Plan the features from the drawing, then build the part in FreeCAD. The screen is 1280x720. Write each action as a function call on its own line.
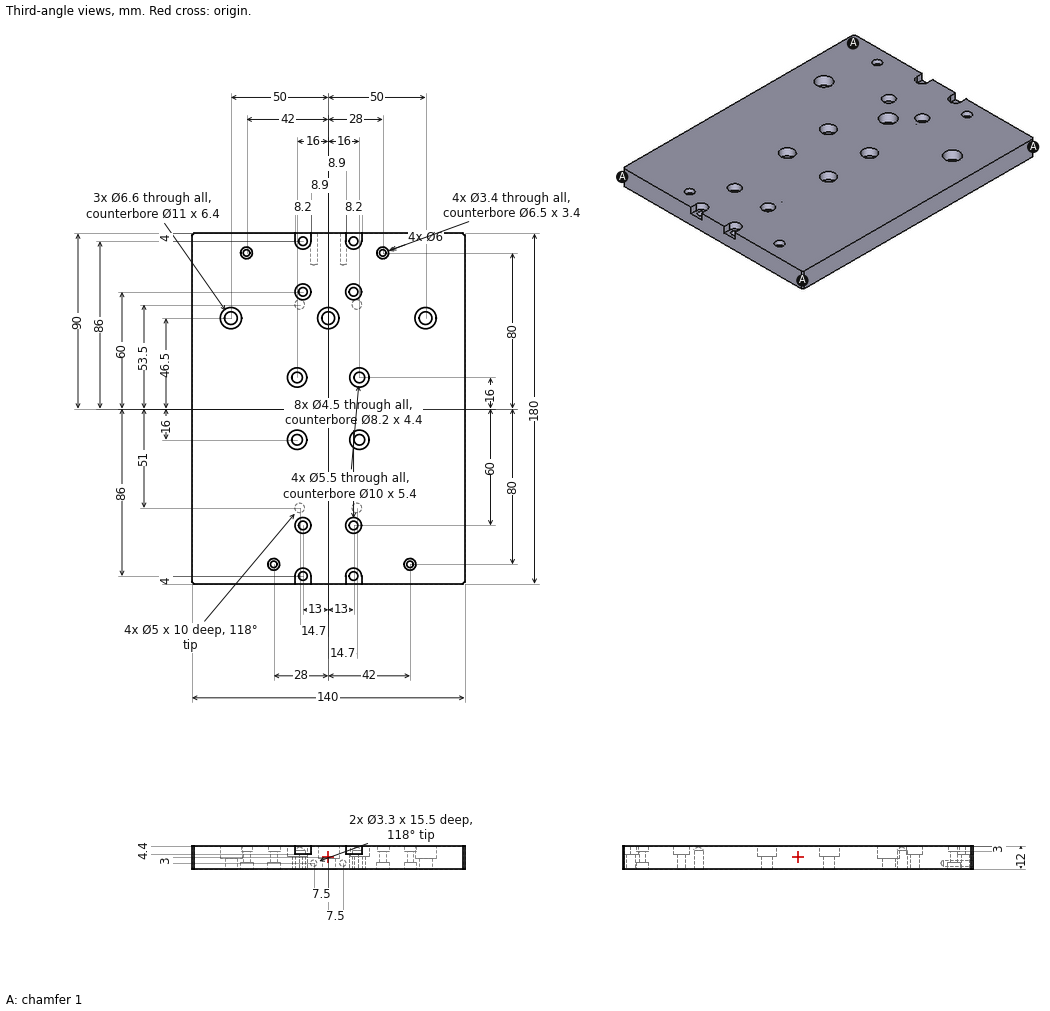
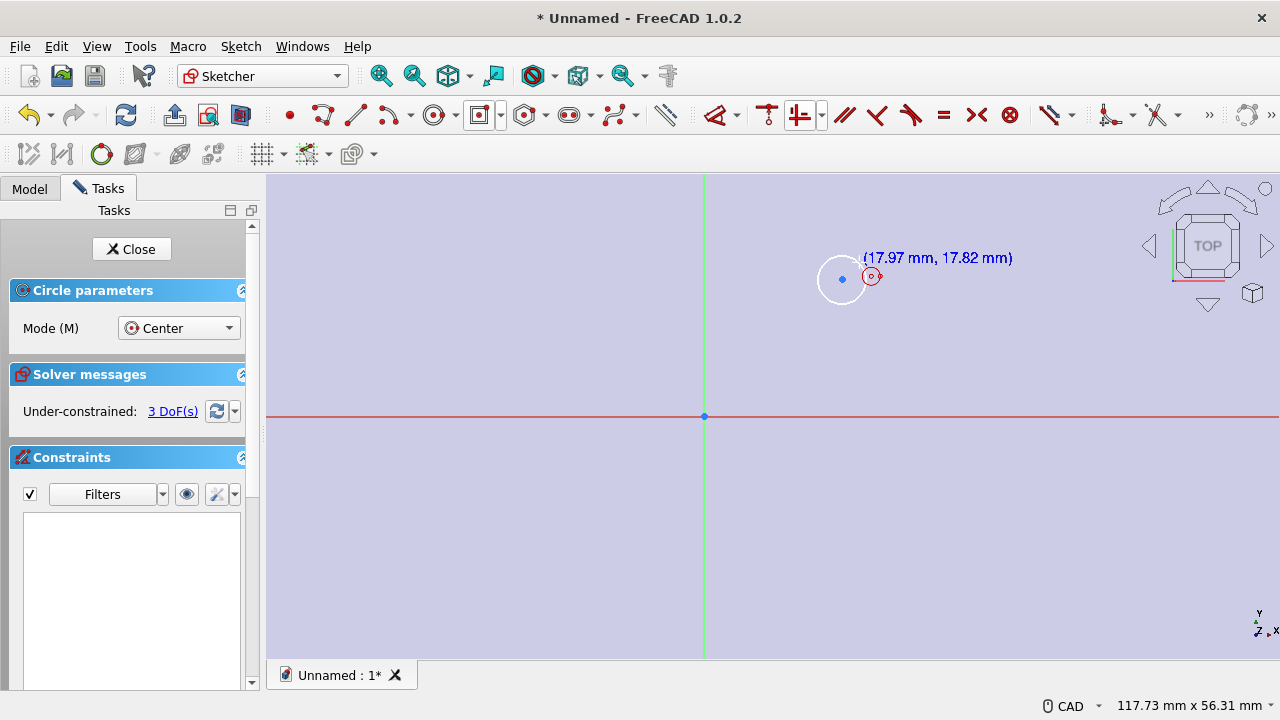
click(566, 279)
click(583, 262)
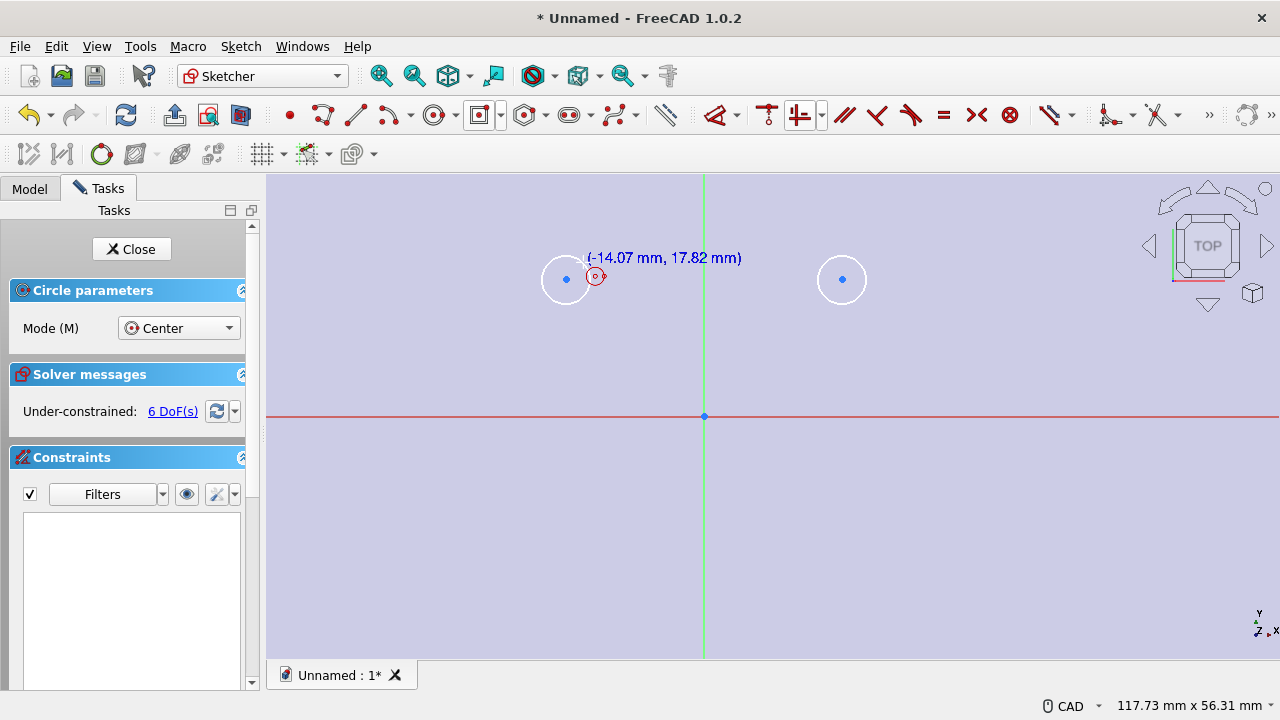
click(566, 554)
click(583, 538)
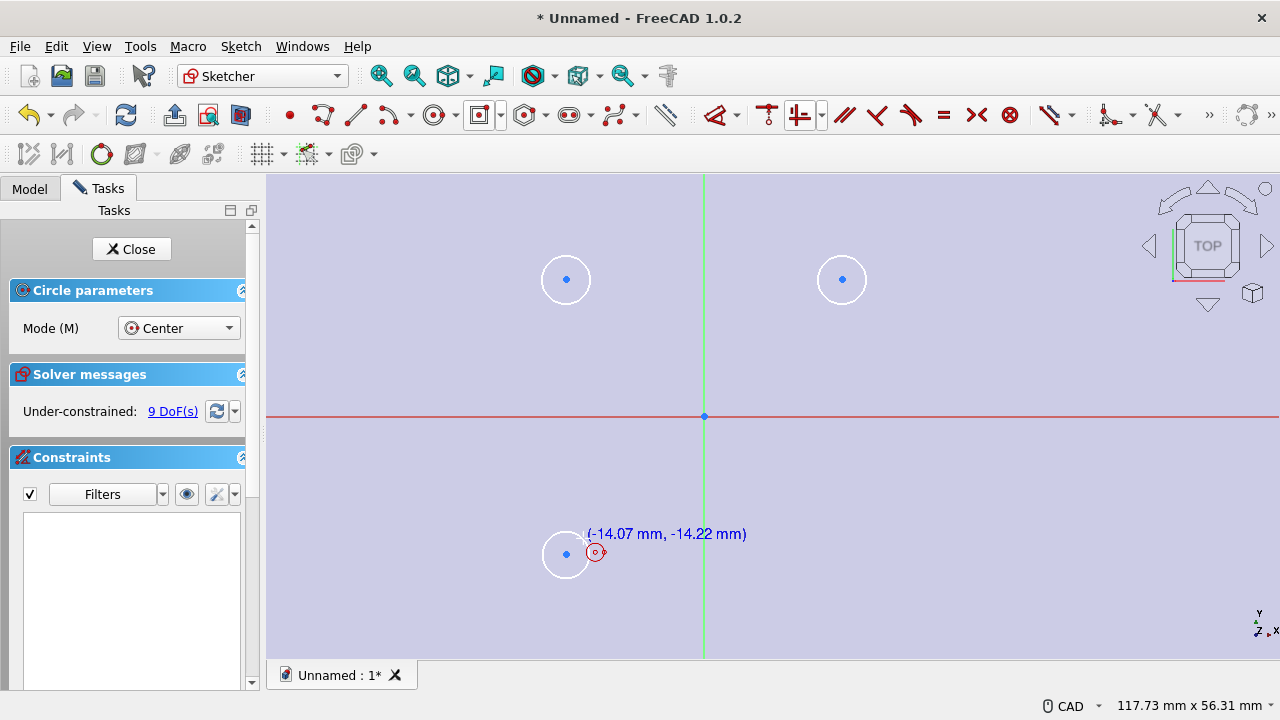
click(842, 554)
click(859, 538)
key(Escape)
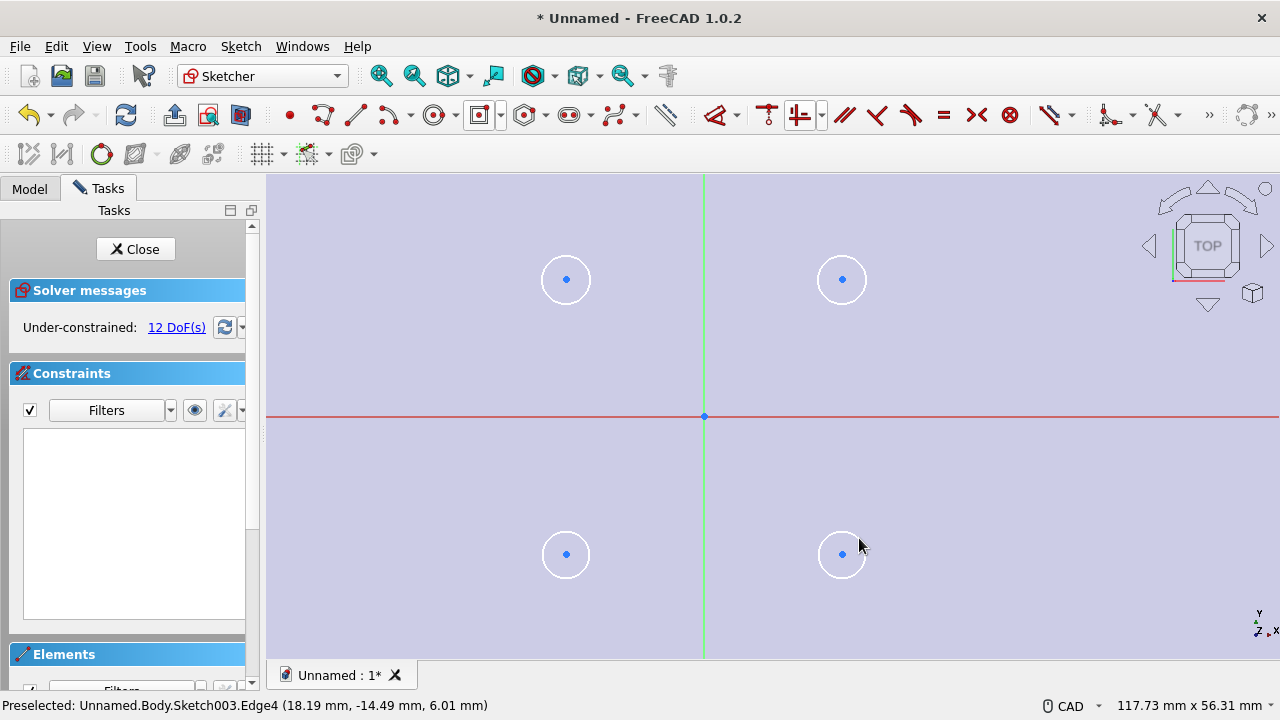
click(859, 263)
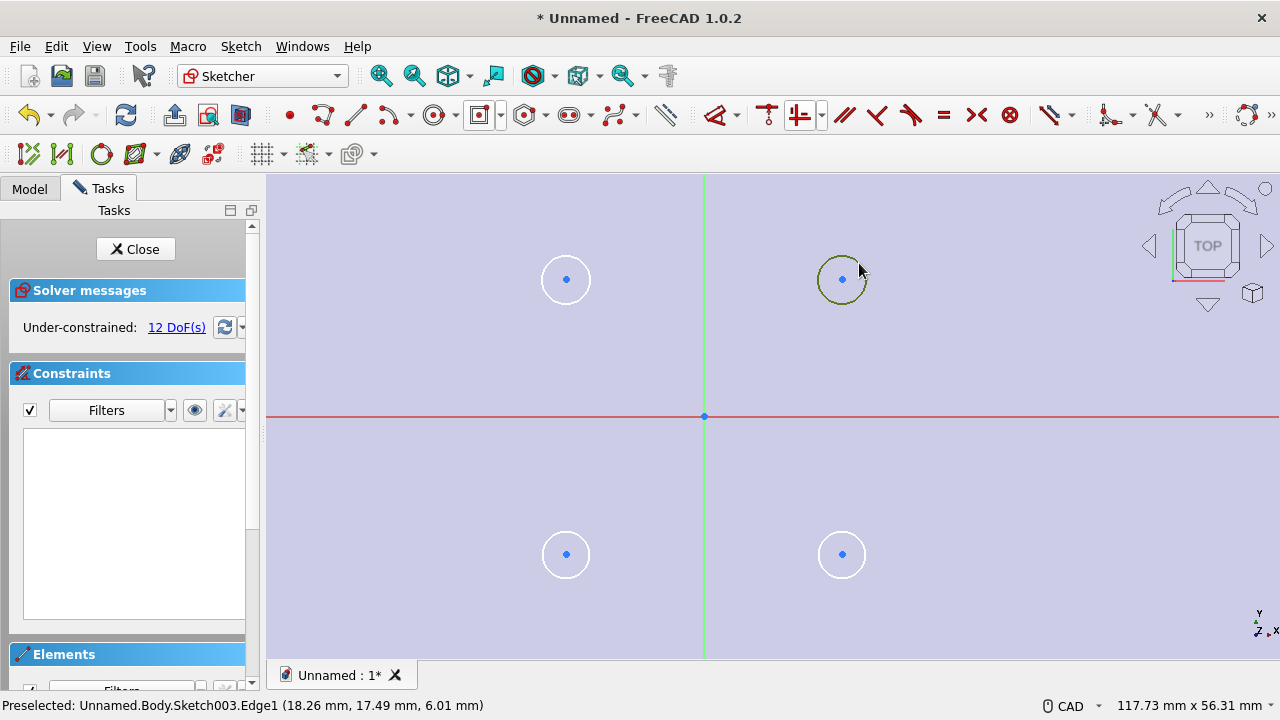
click(583, 263)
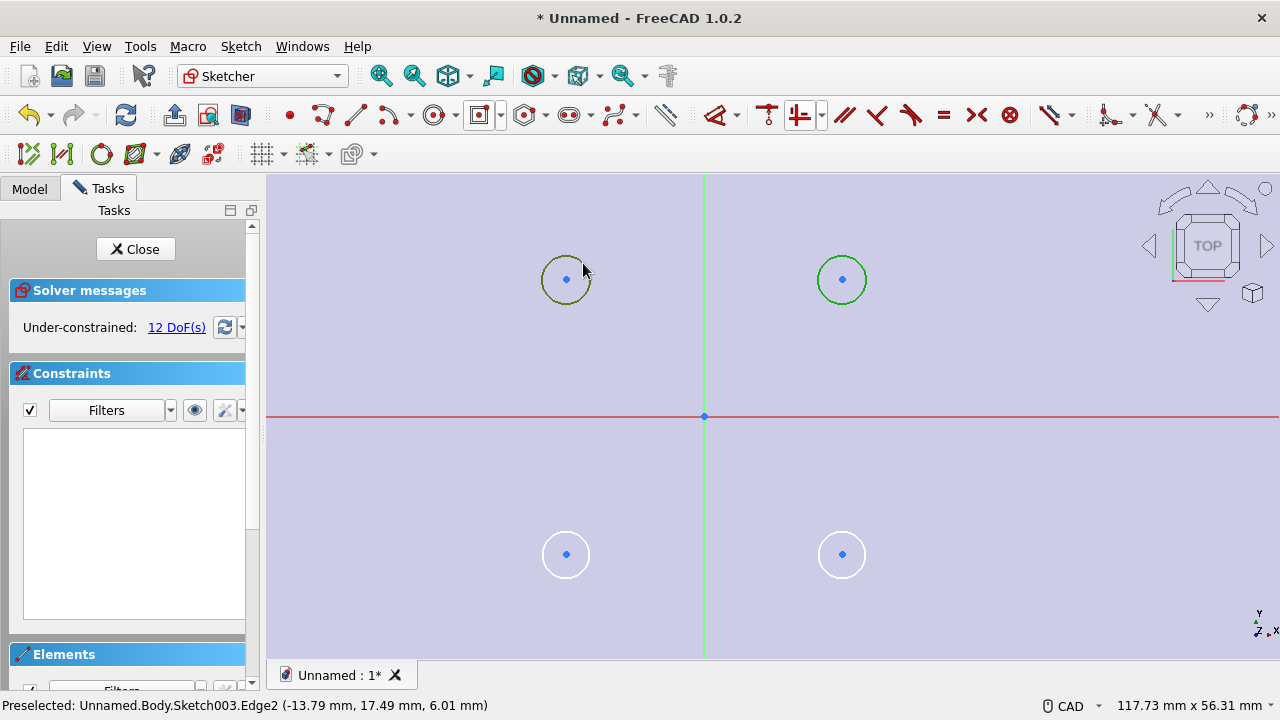
click(582, 538)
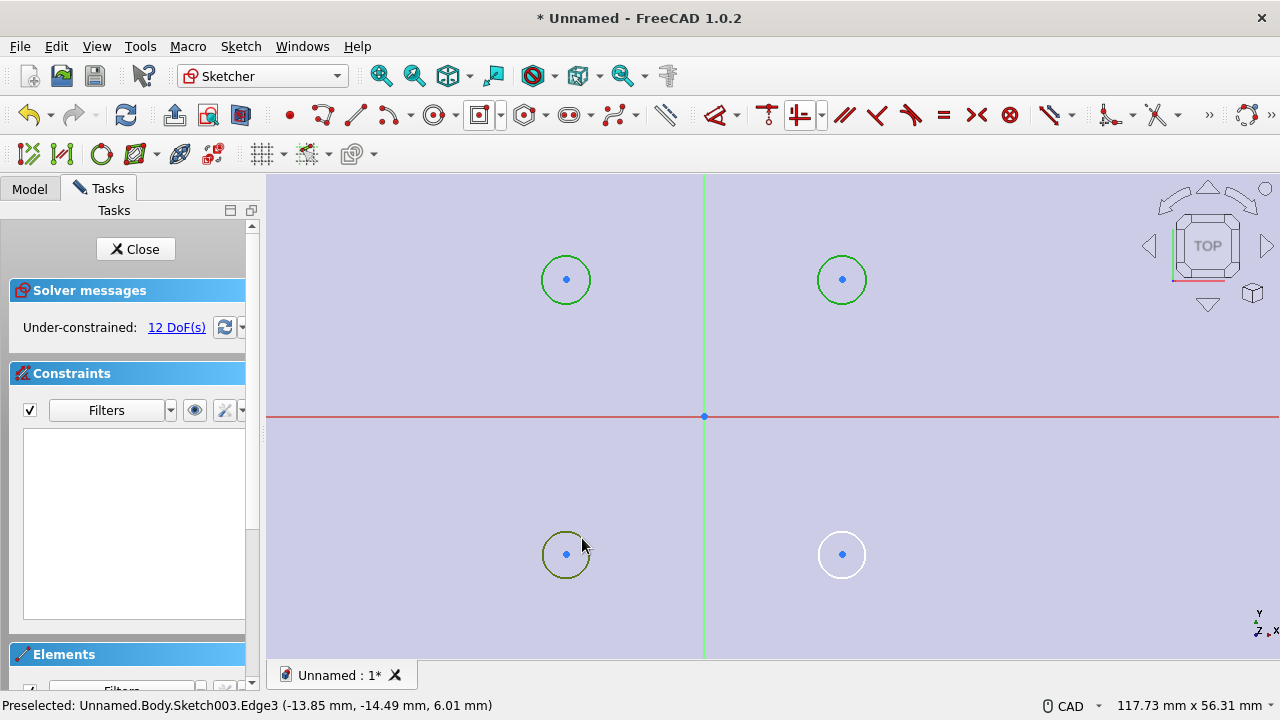
click(858, 538)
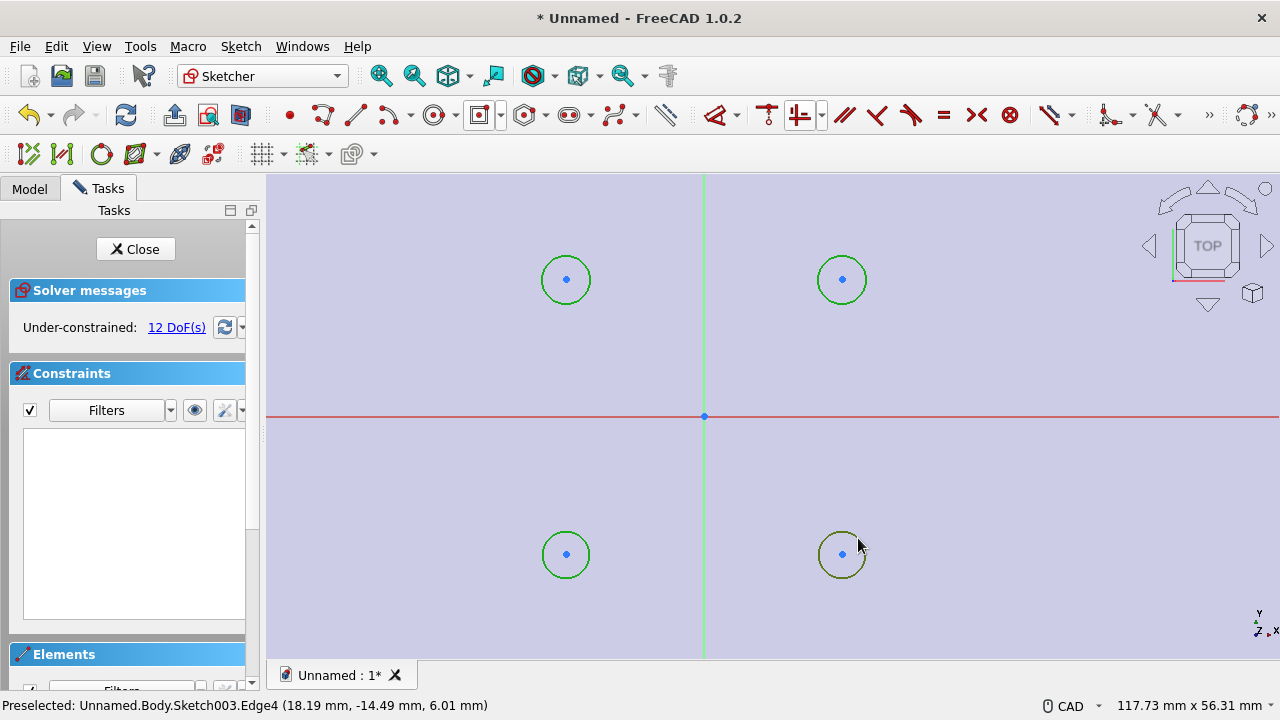
click(944, 116)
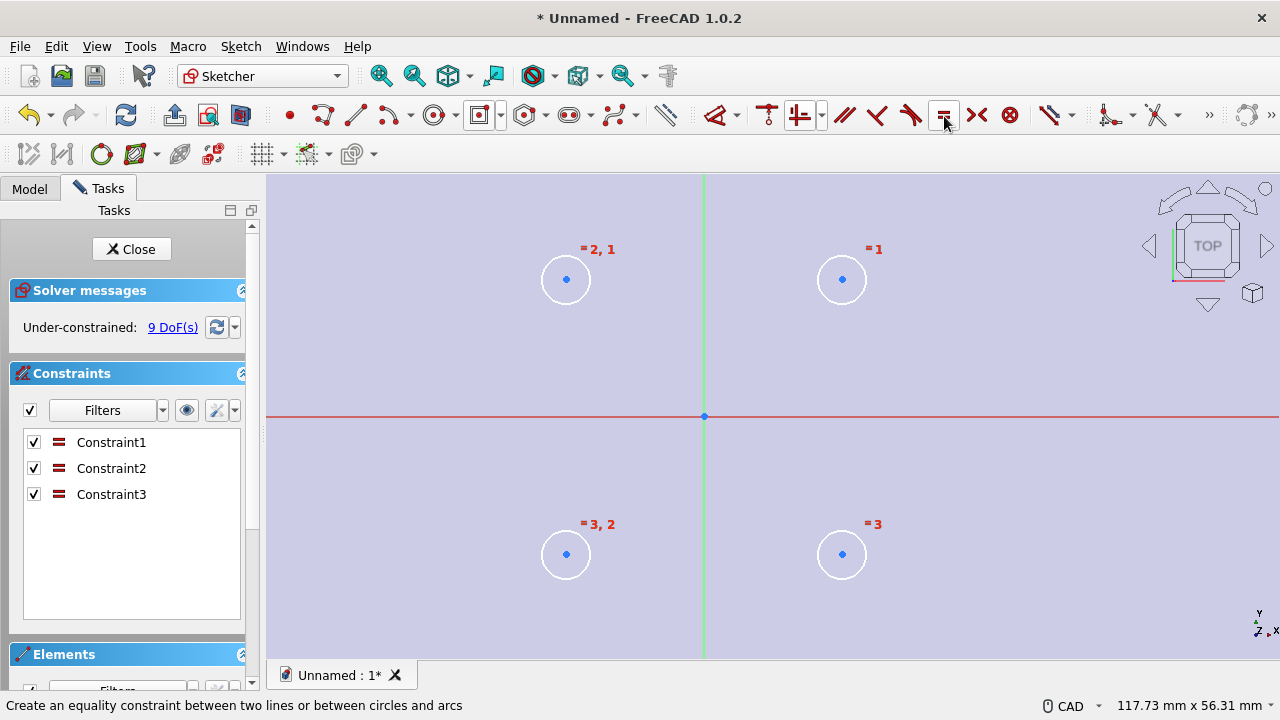
click(714, 116)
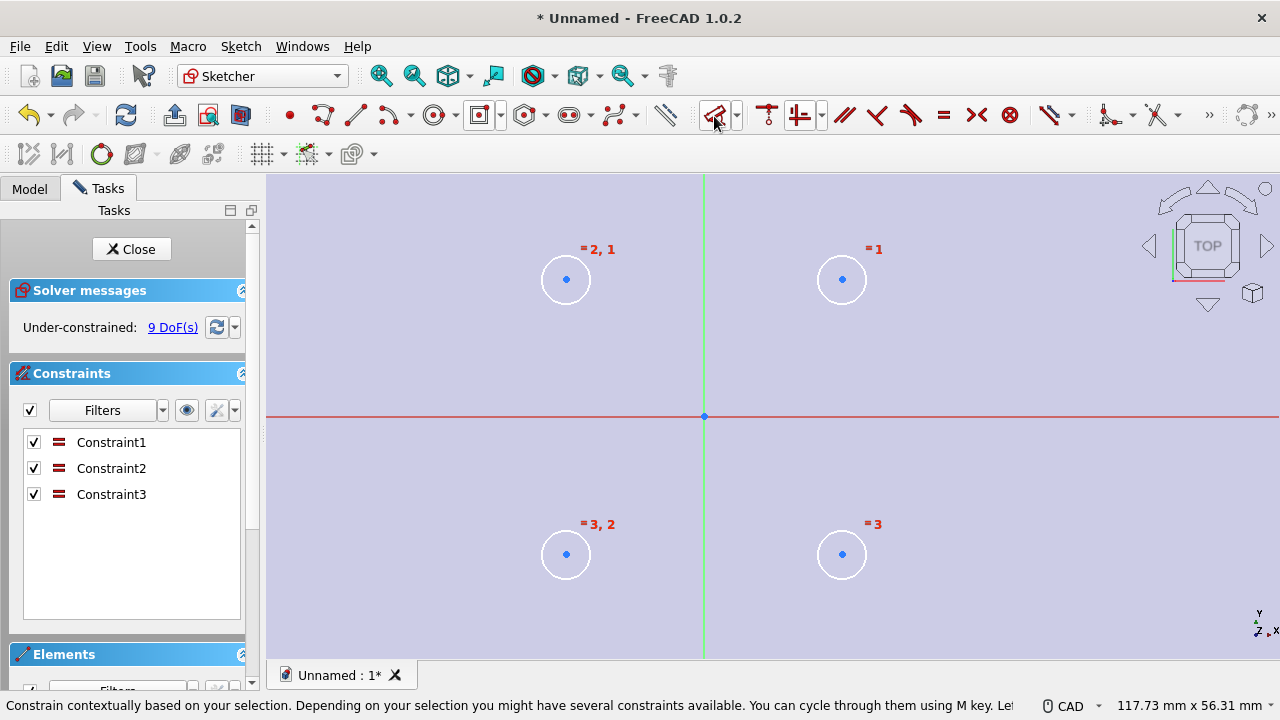
click(859, 263)
click(882, 240)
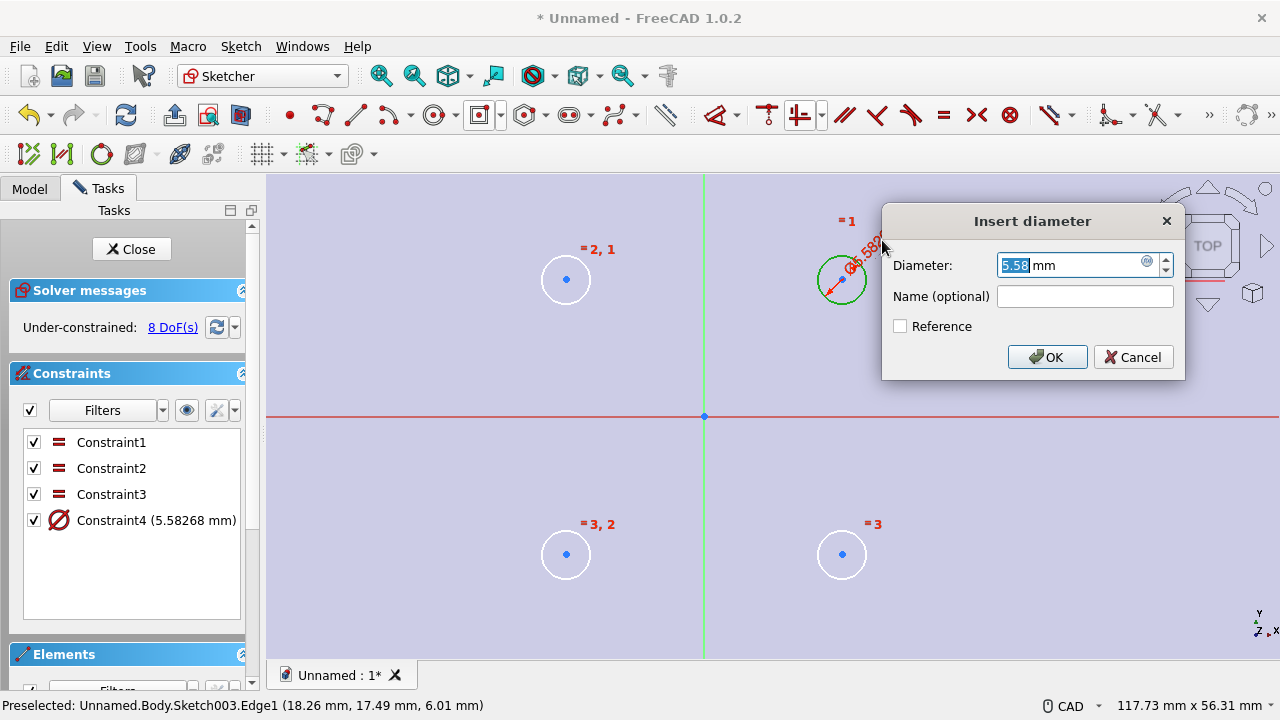
text(5.5)
key(Return)